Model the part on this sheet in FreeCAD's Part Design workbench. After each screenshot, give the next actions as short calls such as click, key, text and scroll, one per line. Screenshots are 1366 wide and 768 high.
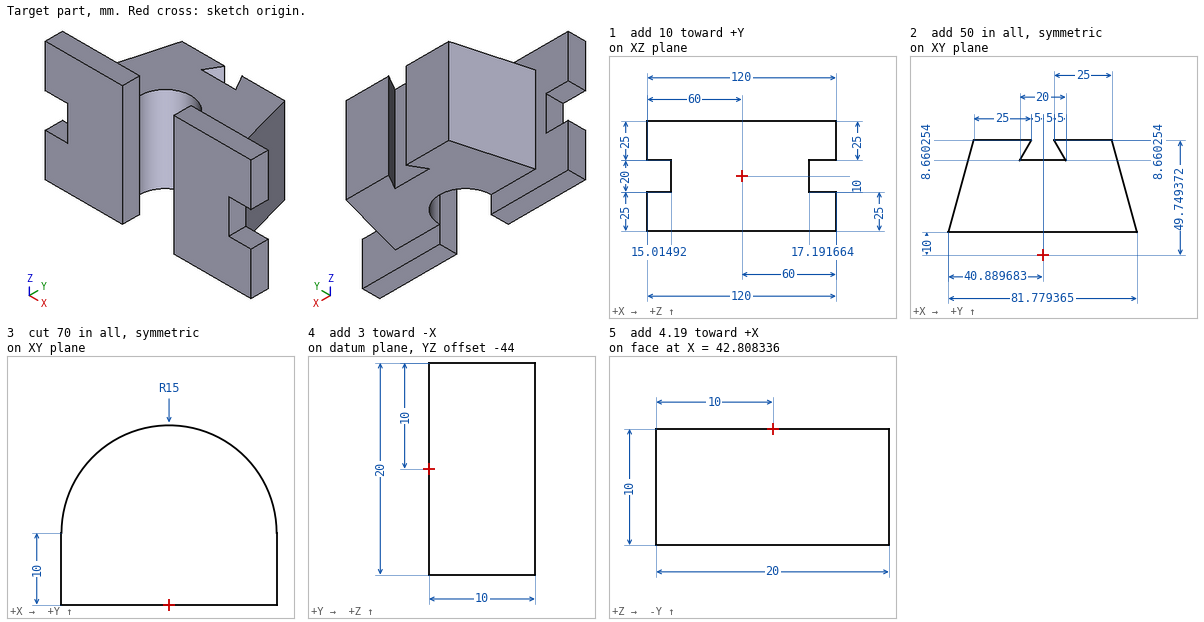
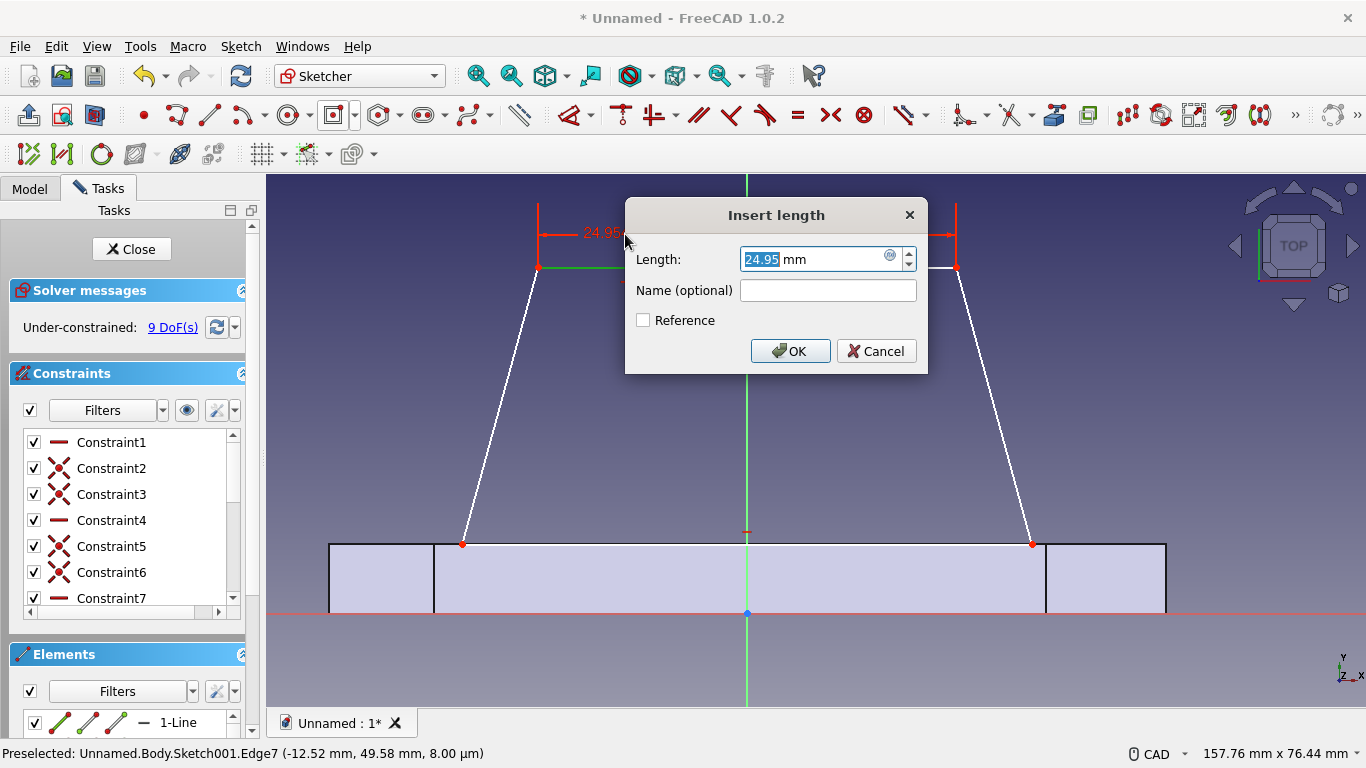
text(25)
key(Return)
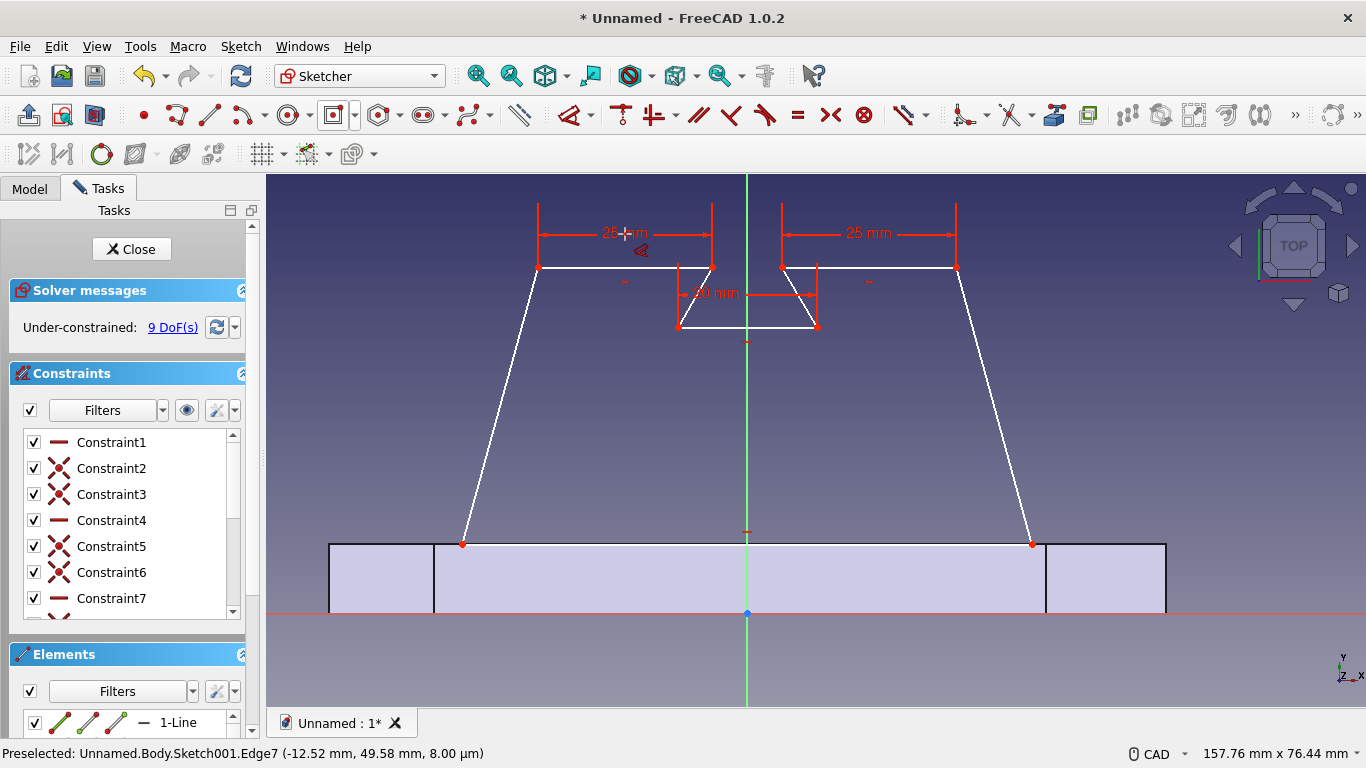
click(782, 268)
click(765, 648)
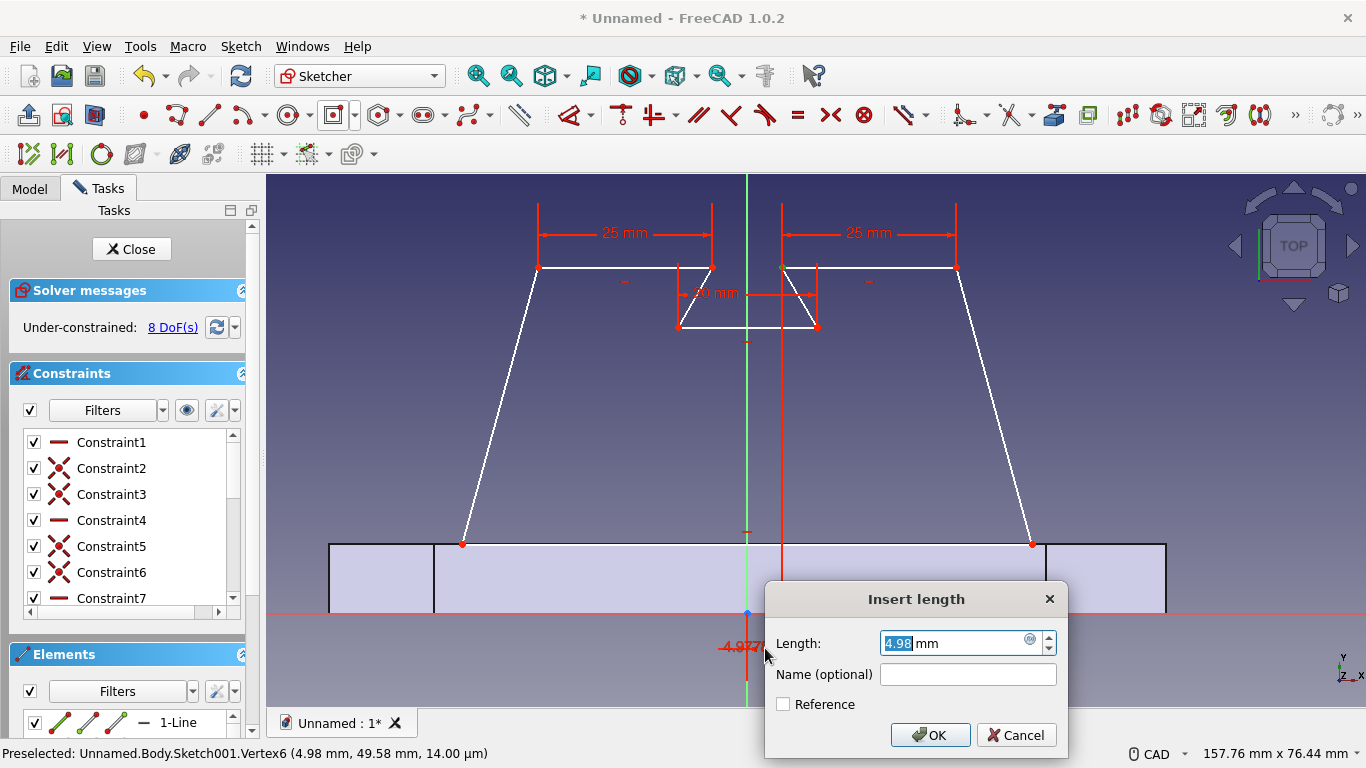
text(5)
key(Return)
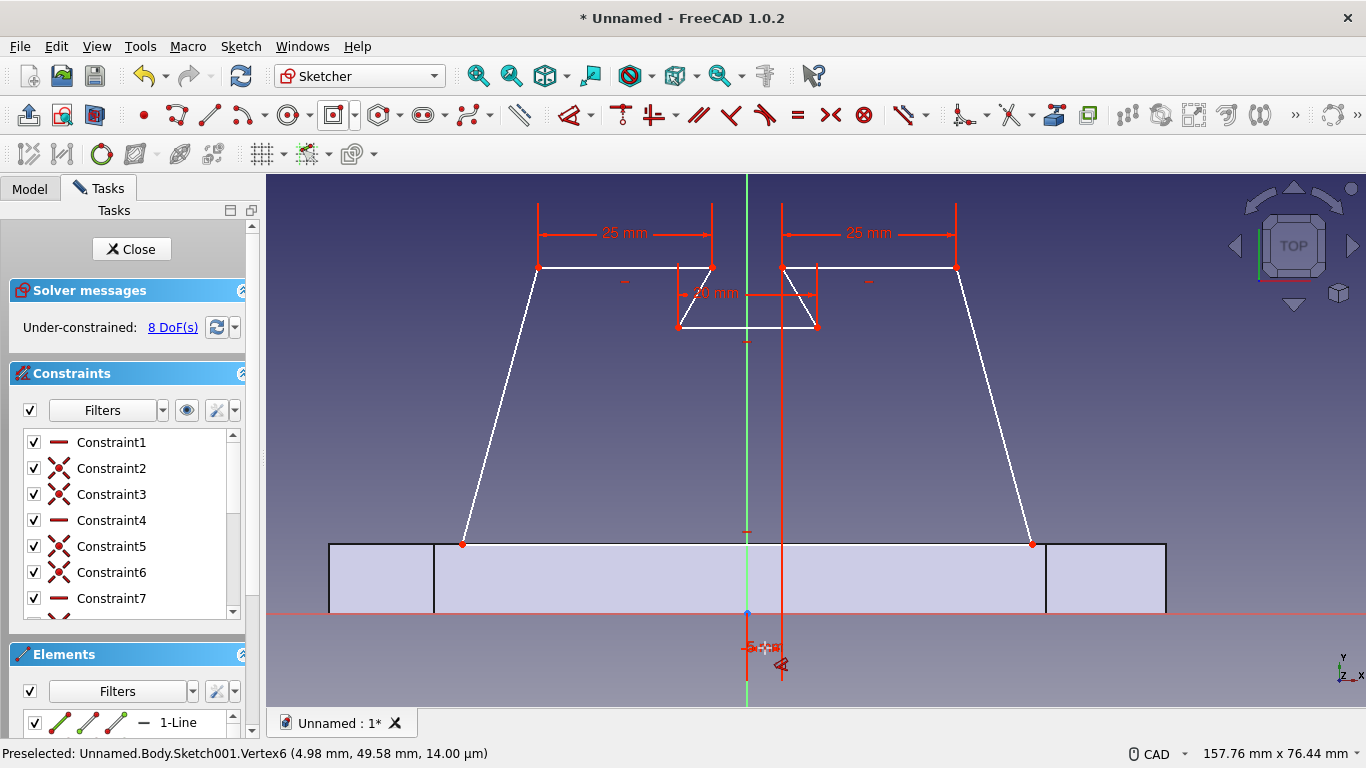
click(712, 268)
click(730, 234)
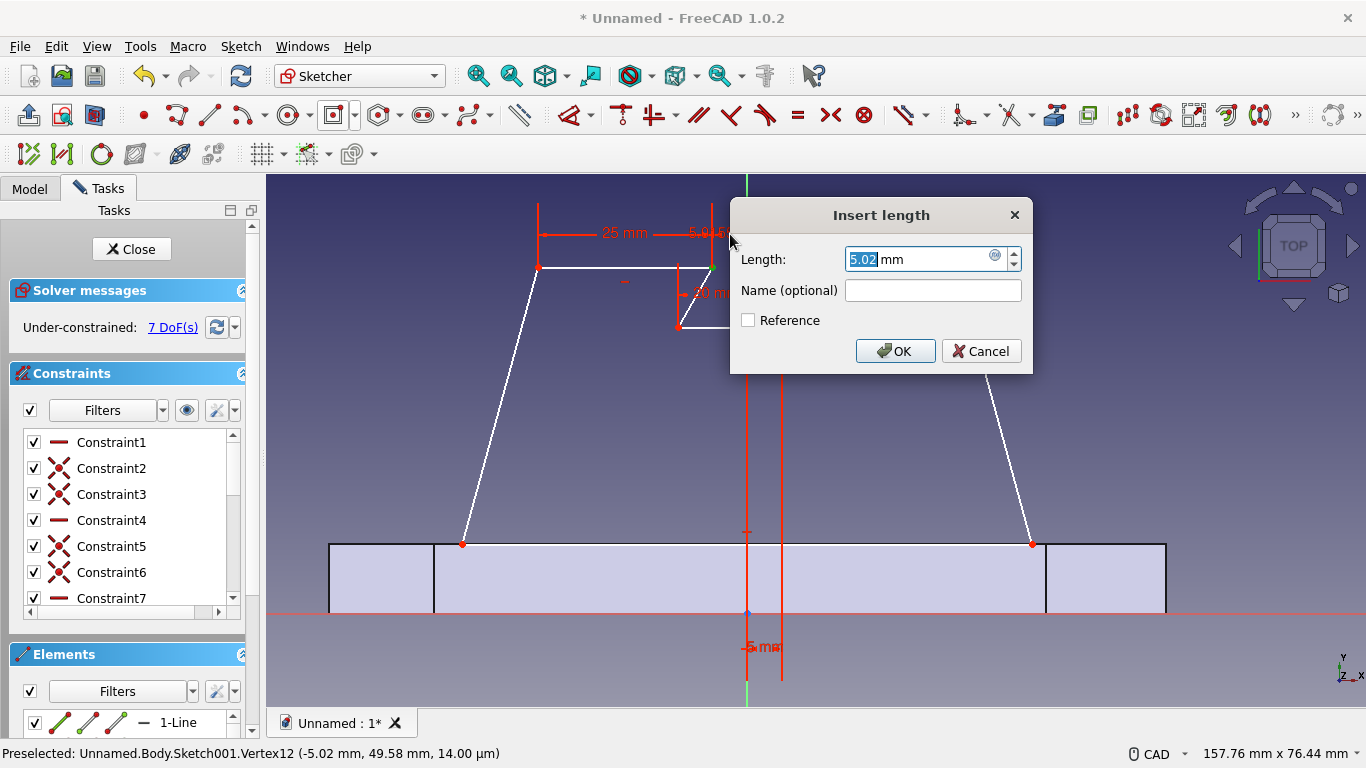
text(5)
key(Return)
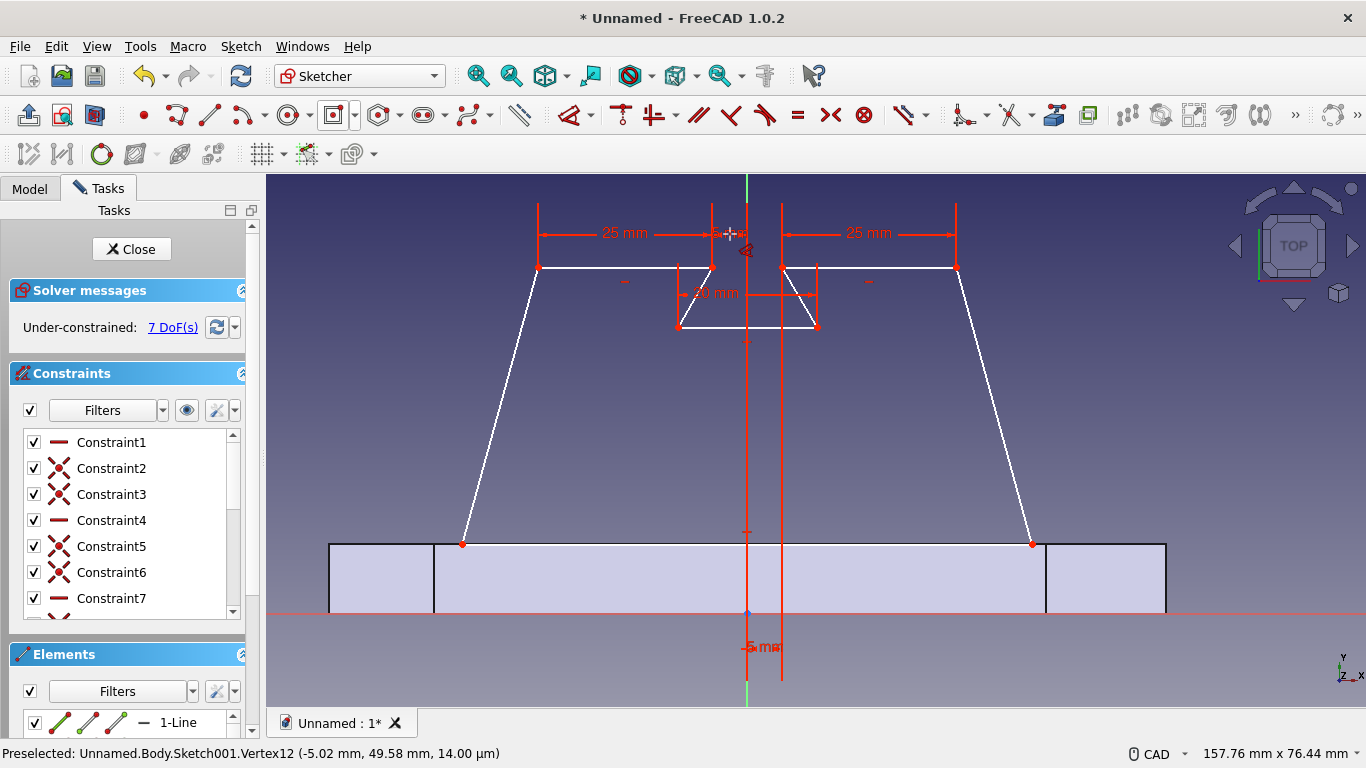
click(793, 286)
click(800, 362)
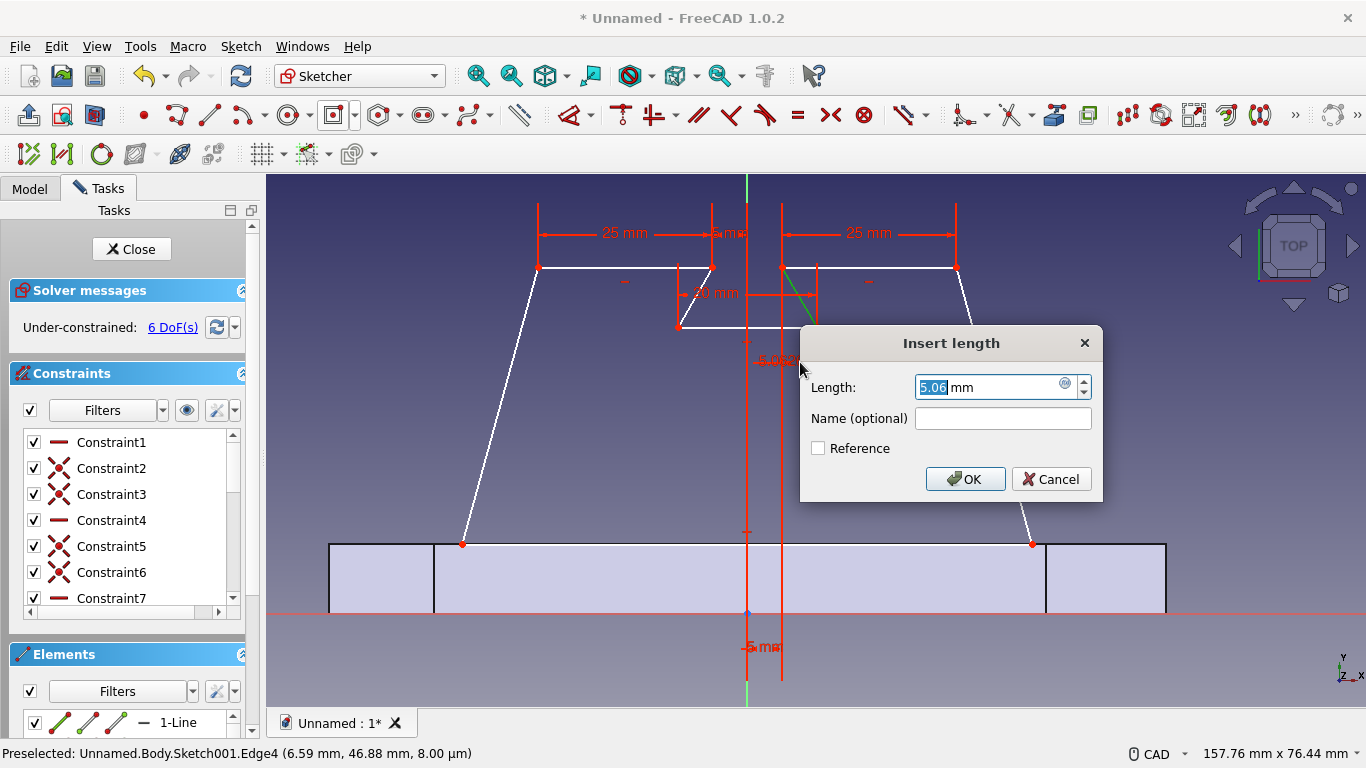
text(5)
key(Return)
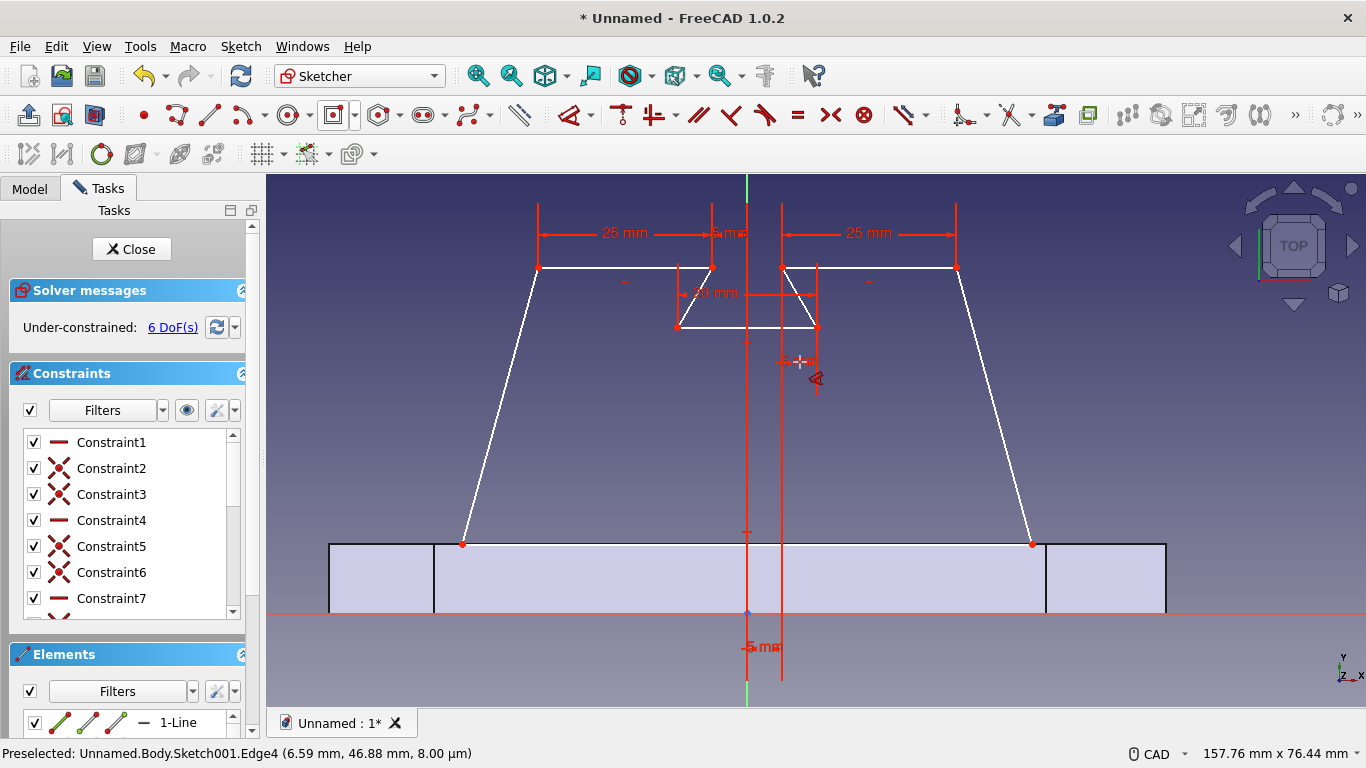
click(462, 545)
click(428, 579)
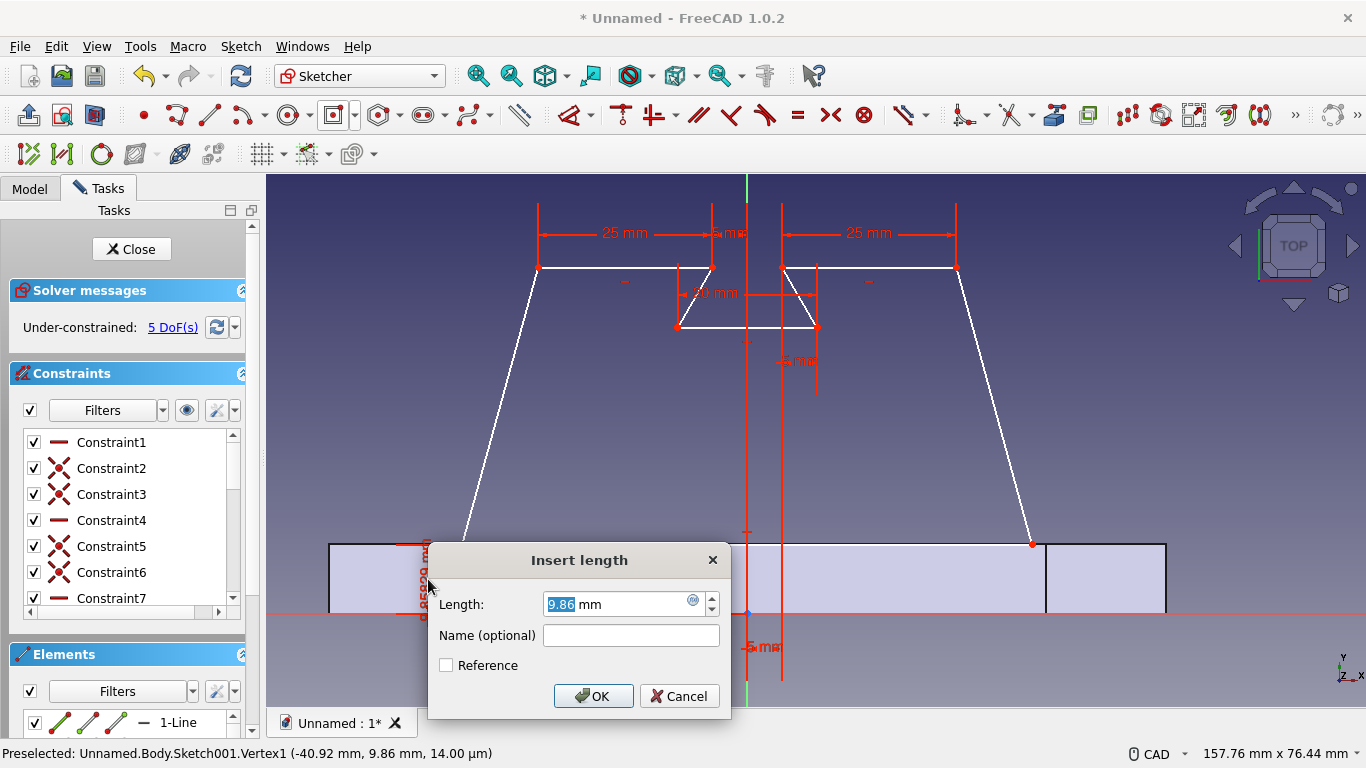
text(10)
key(Return)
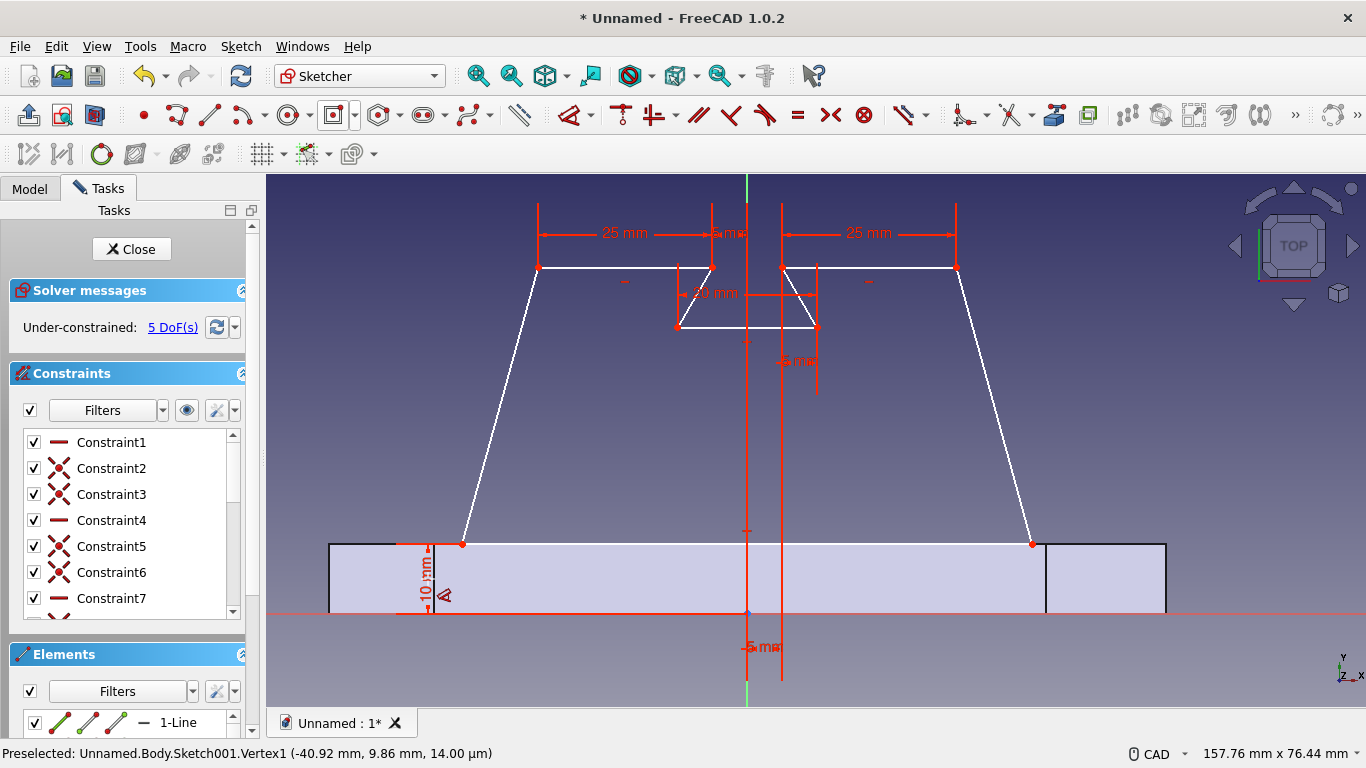
click(633, 544)
click(616, 578)